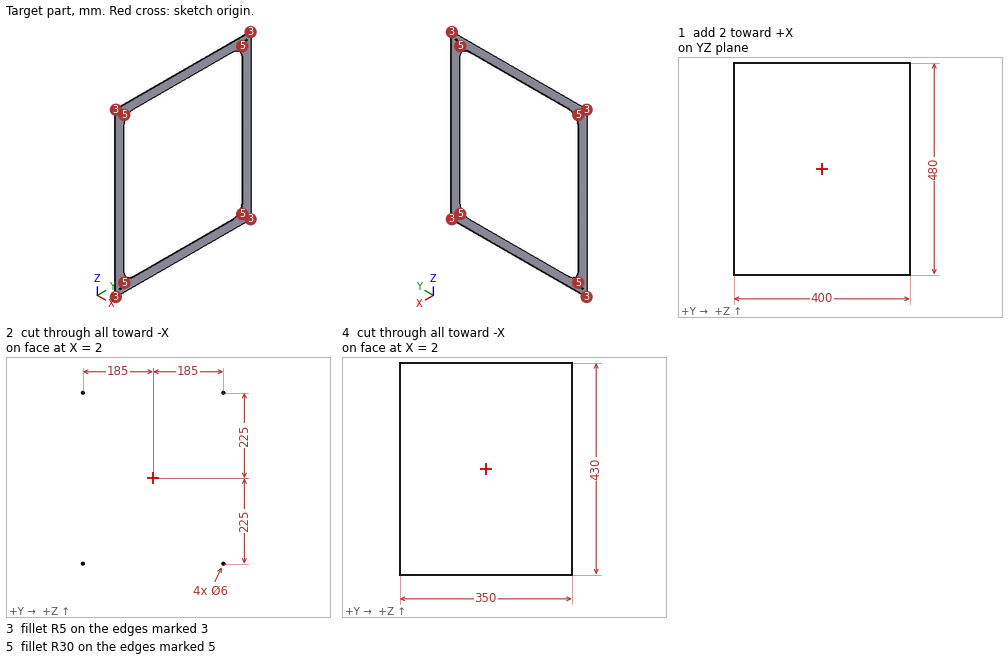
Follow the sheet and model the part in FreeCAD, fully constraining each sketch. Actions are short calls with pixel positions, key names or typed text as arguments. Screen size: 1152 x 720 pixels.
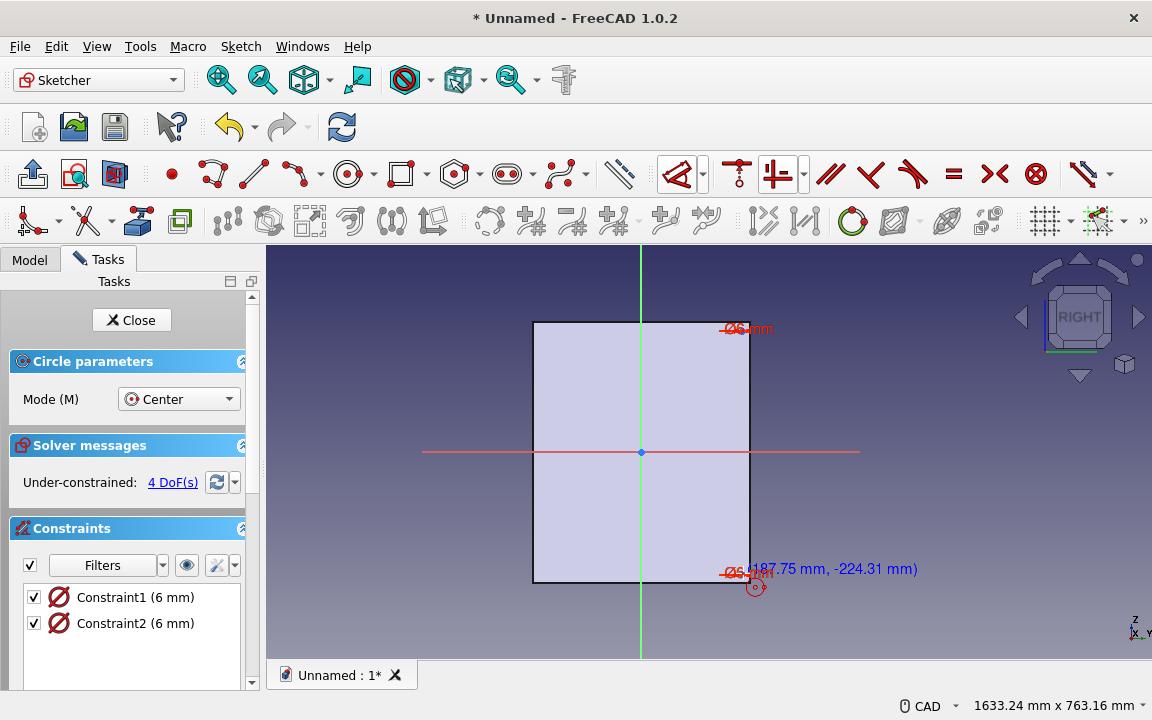
scroll(541, 330, up, 14)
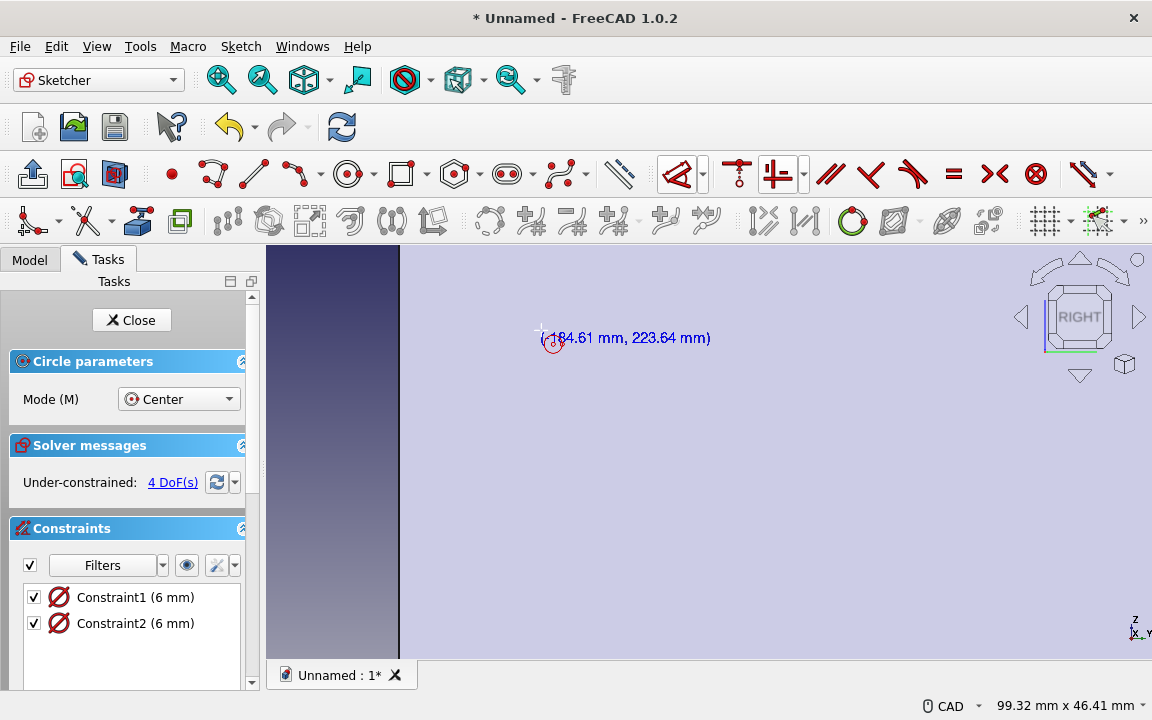
scroll(541, 330, down, 14)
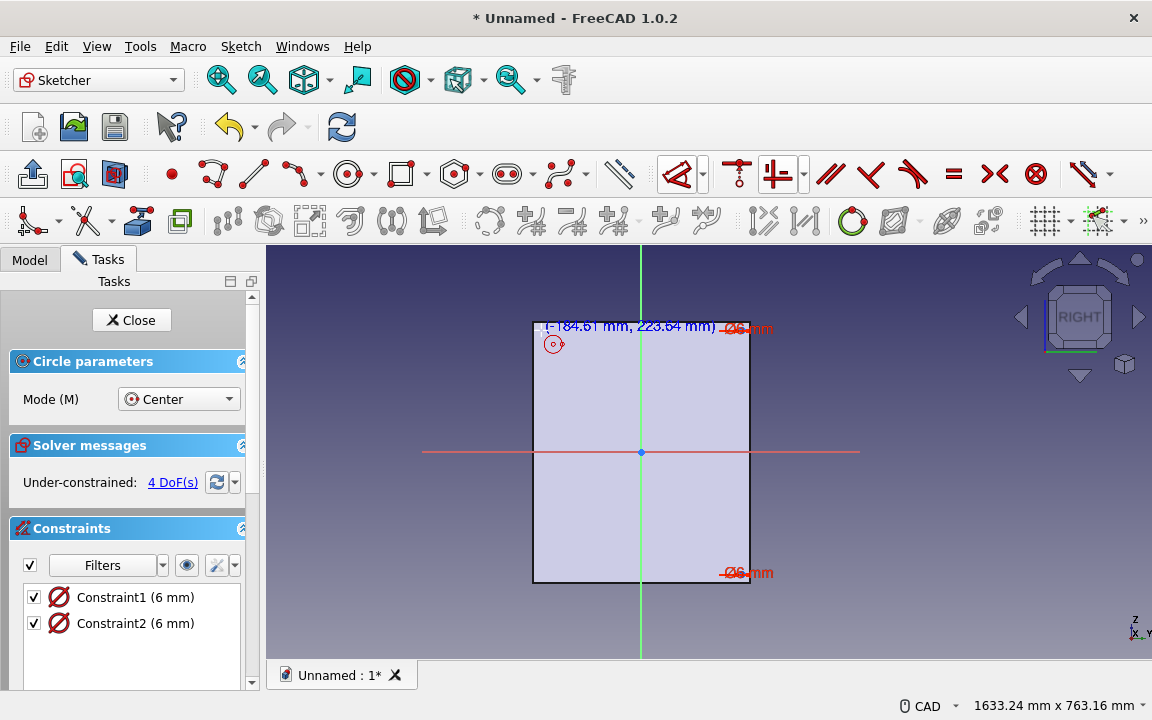
click(541, 330)
move(542, 329)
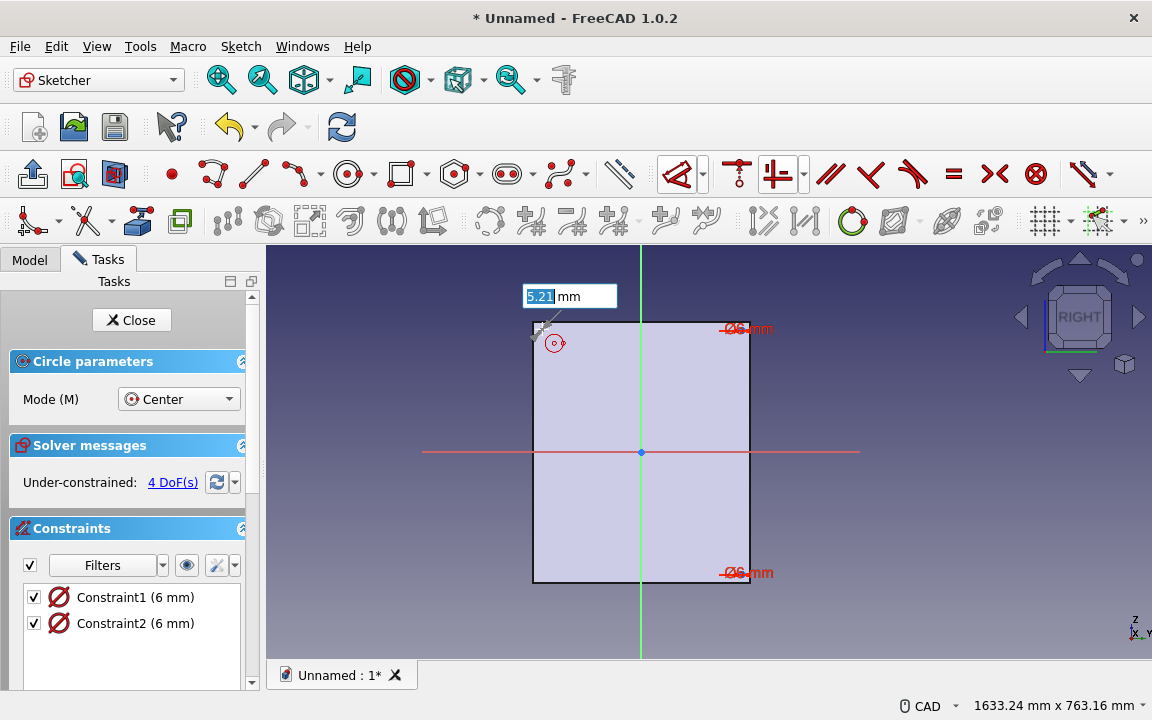
text(6)
key(Return)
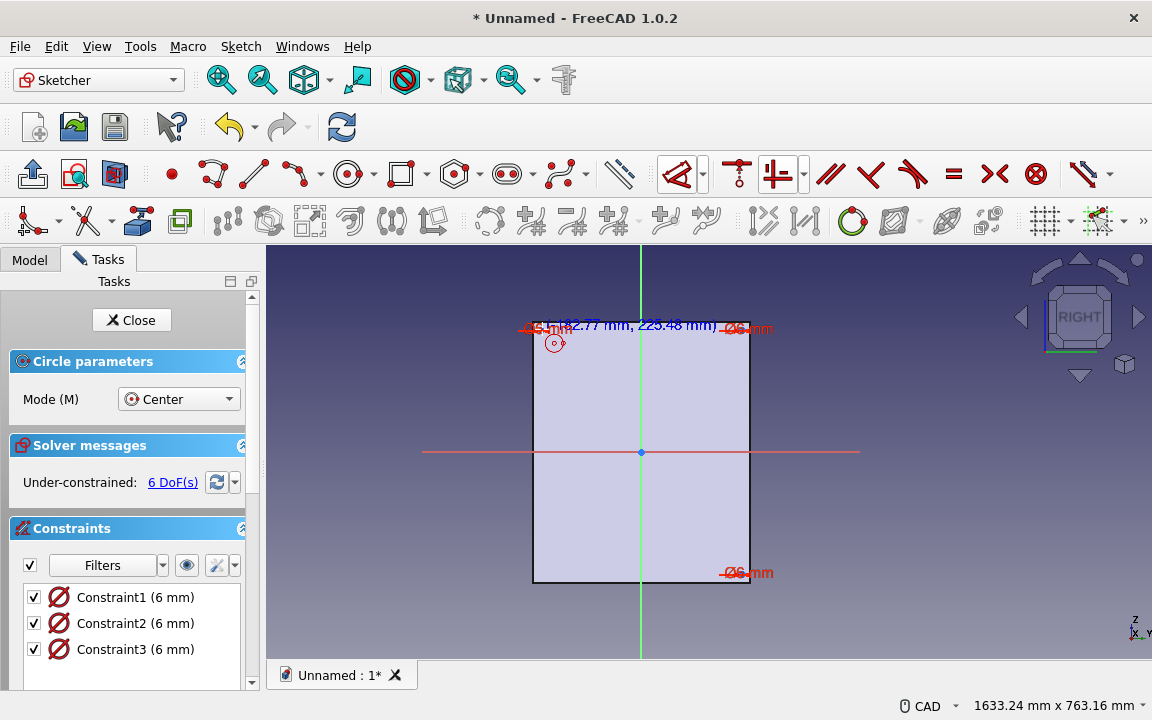
scroll(541, 574, up, 14)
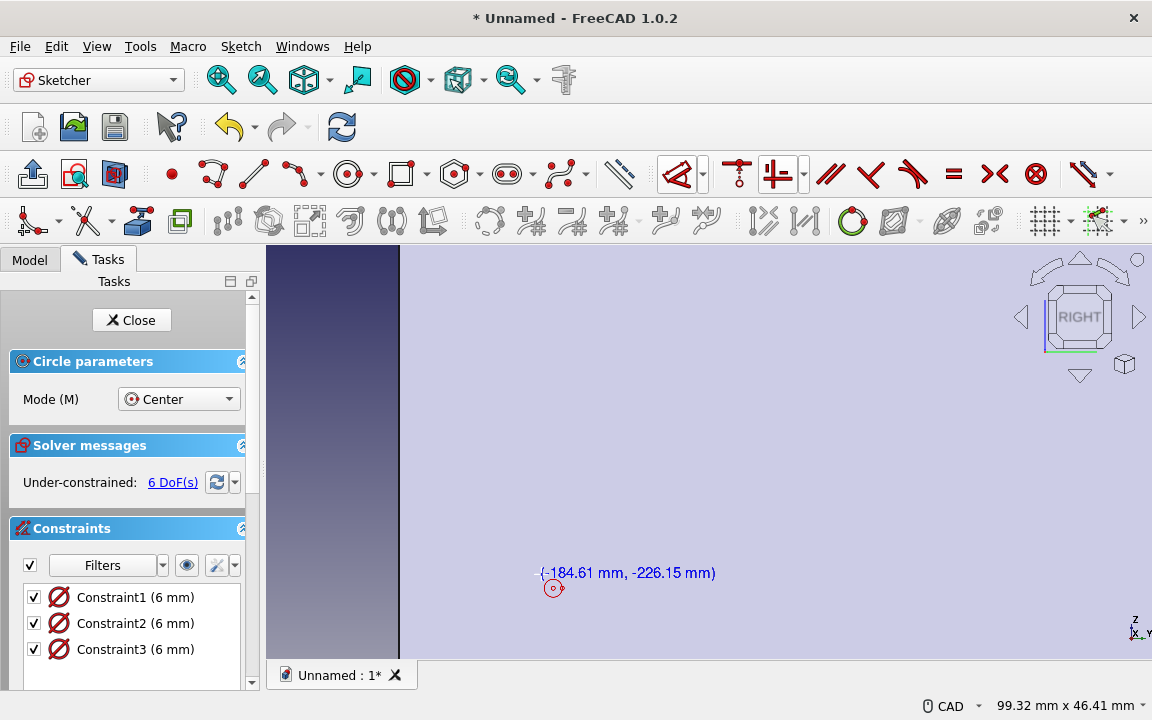
scroll(541, 574, down, 14)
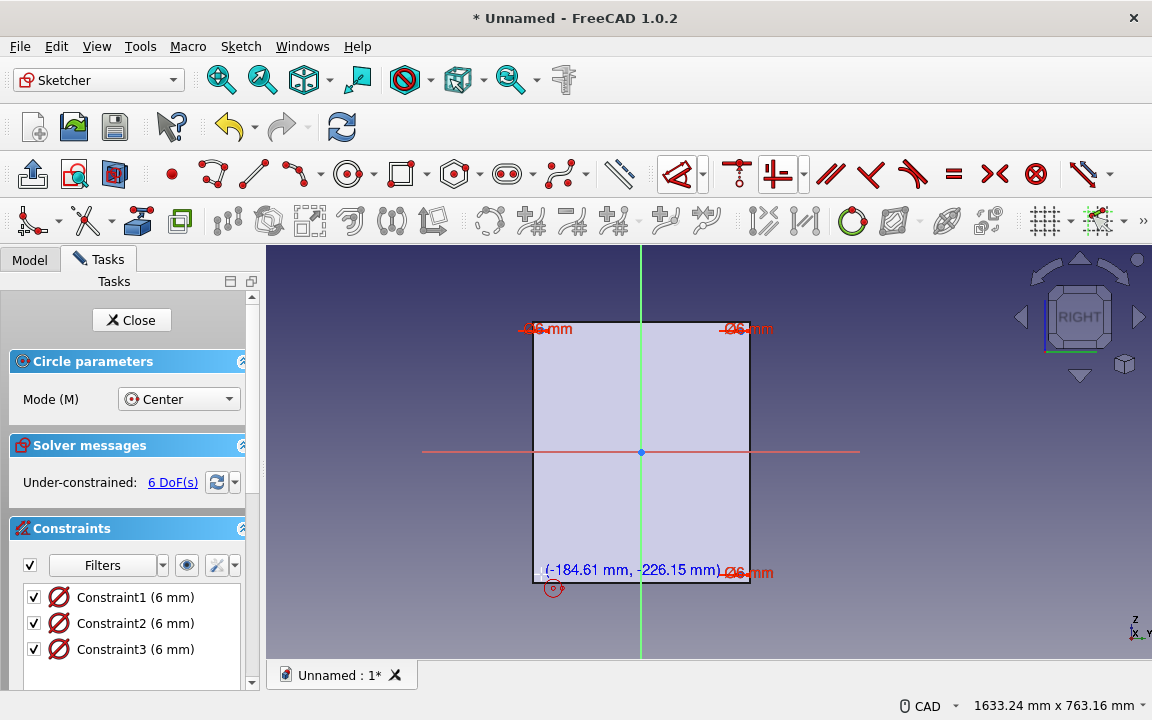
click(541, 574)
move(542, 573)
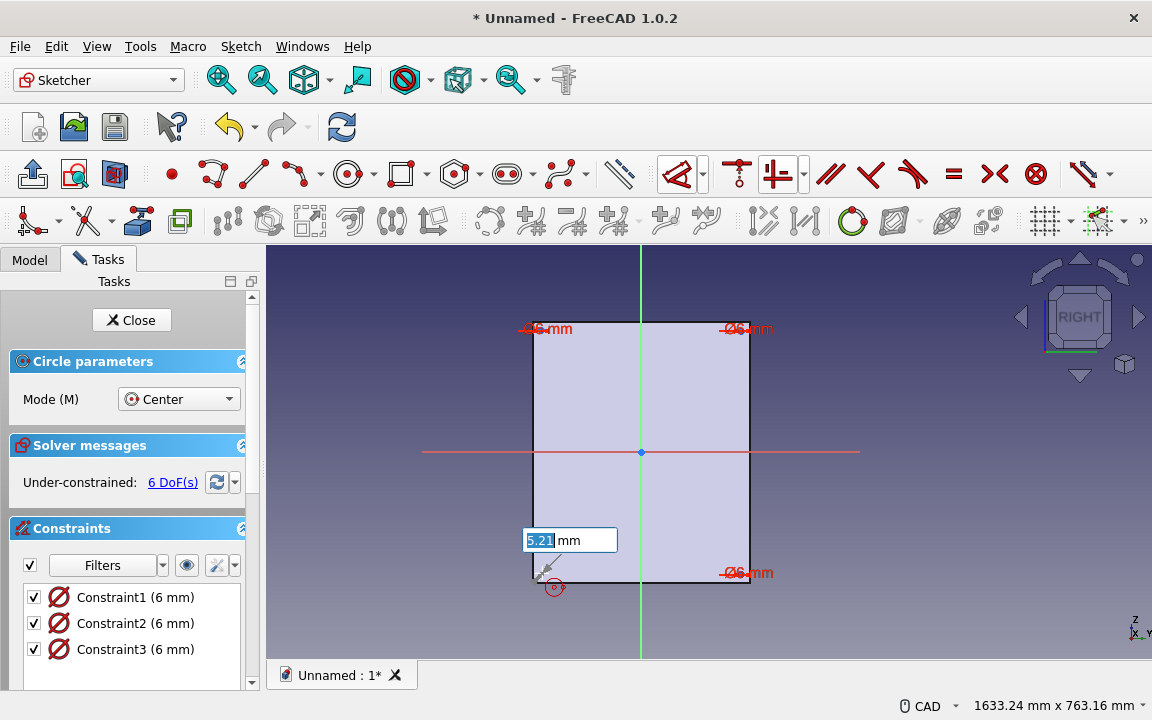
text(6)
key(Return)
key(Escape)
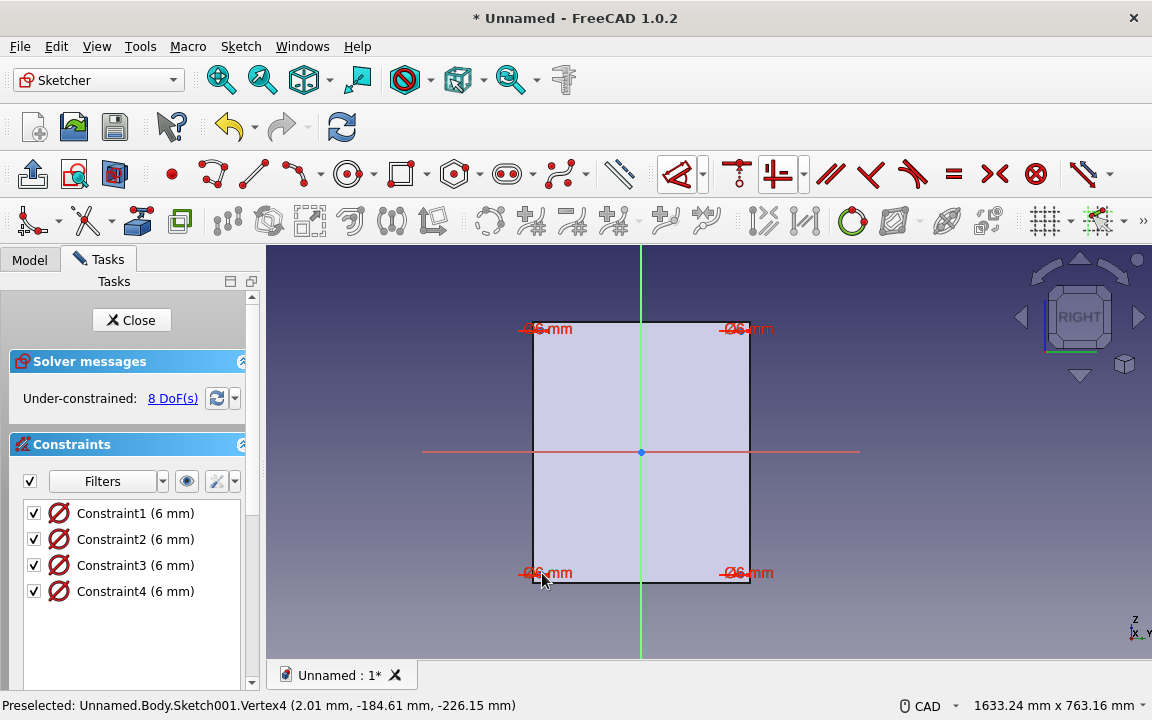
click(742, 331)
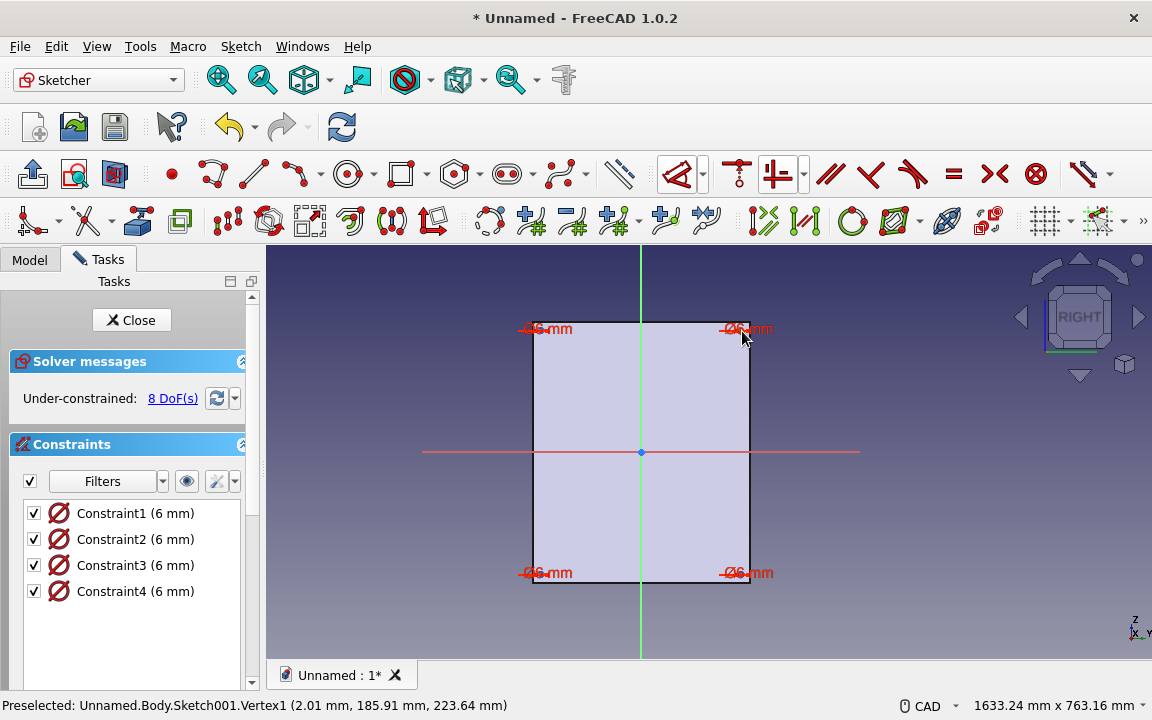
click(742, 575)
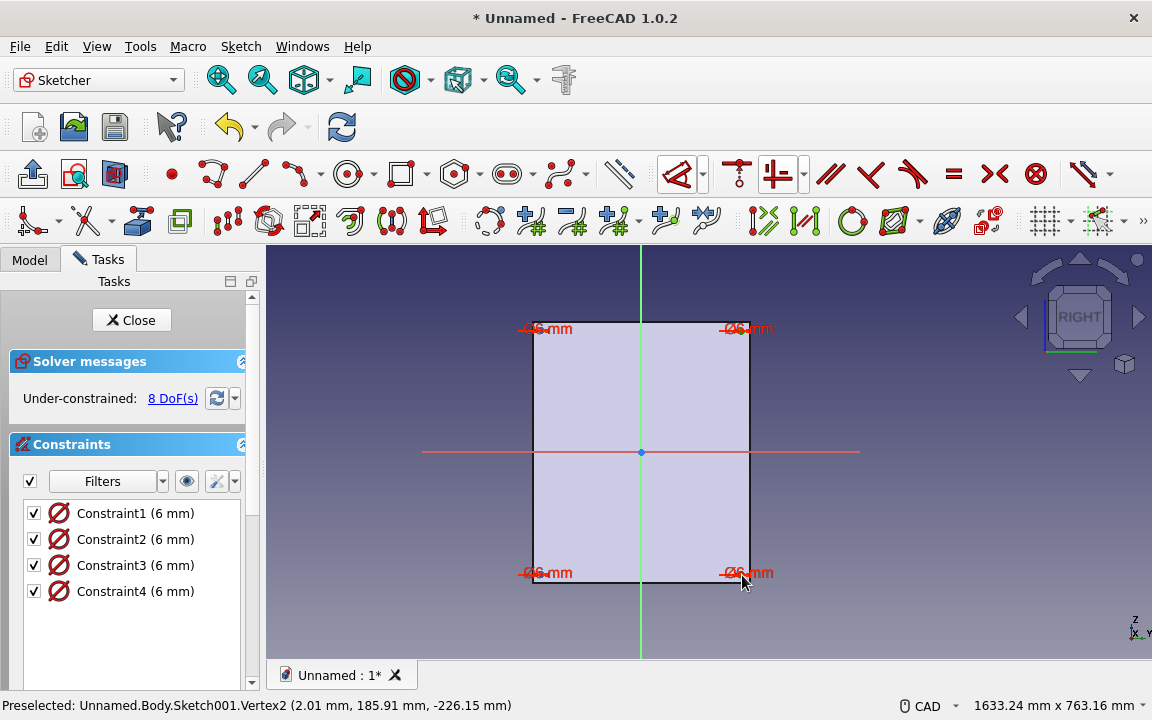
key(v)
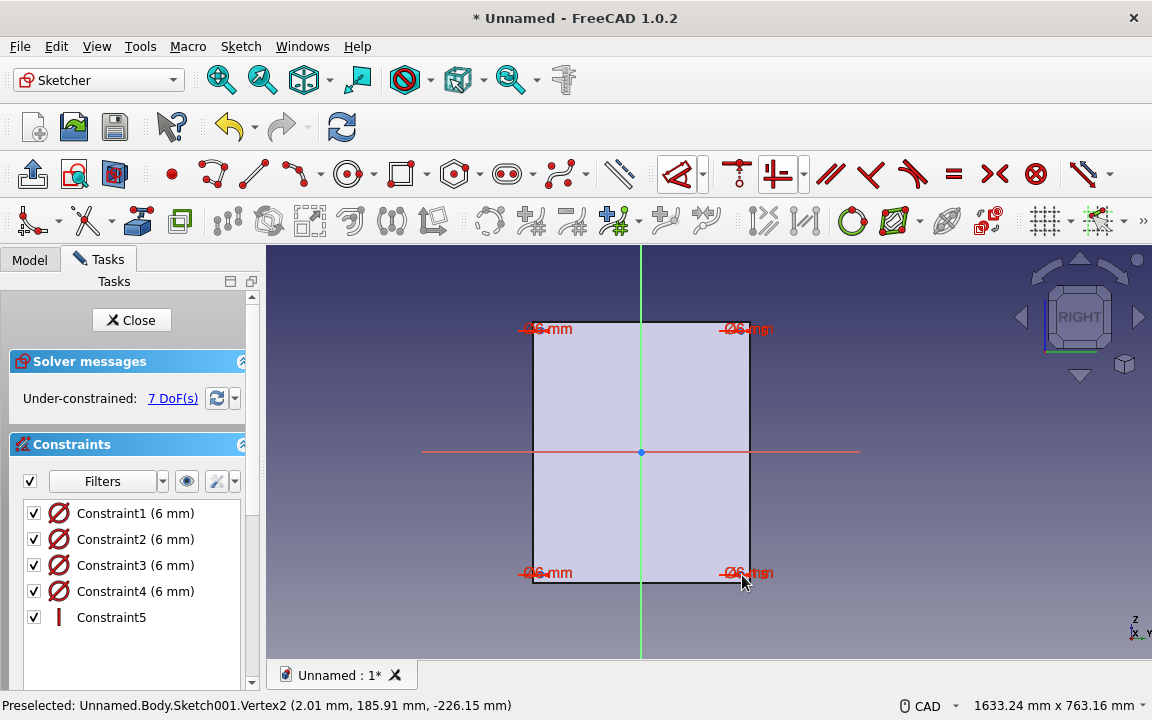
click(742, 331)